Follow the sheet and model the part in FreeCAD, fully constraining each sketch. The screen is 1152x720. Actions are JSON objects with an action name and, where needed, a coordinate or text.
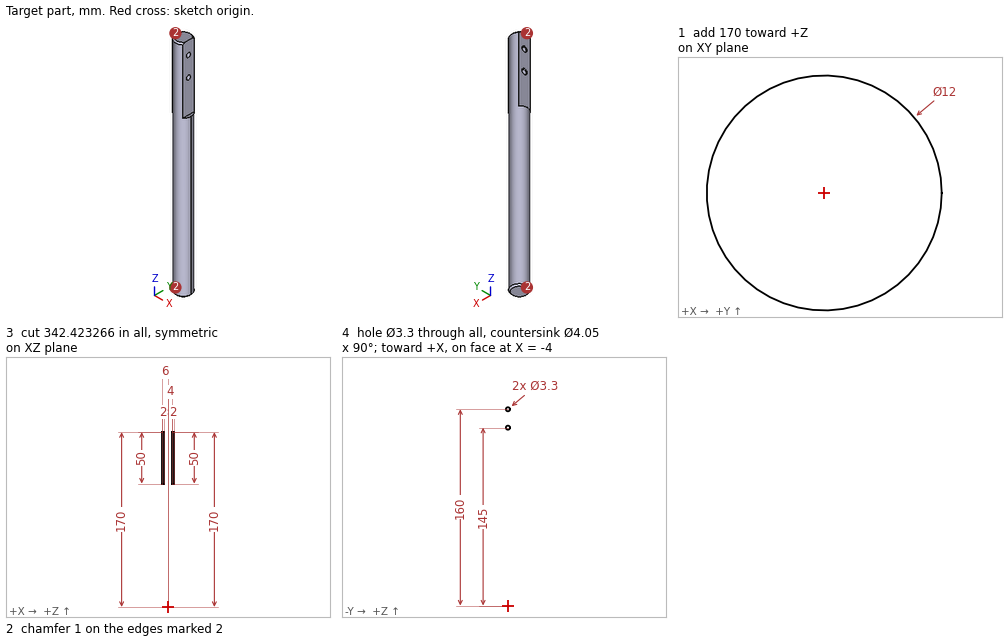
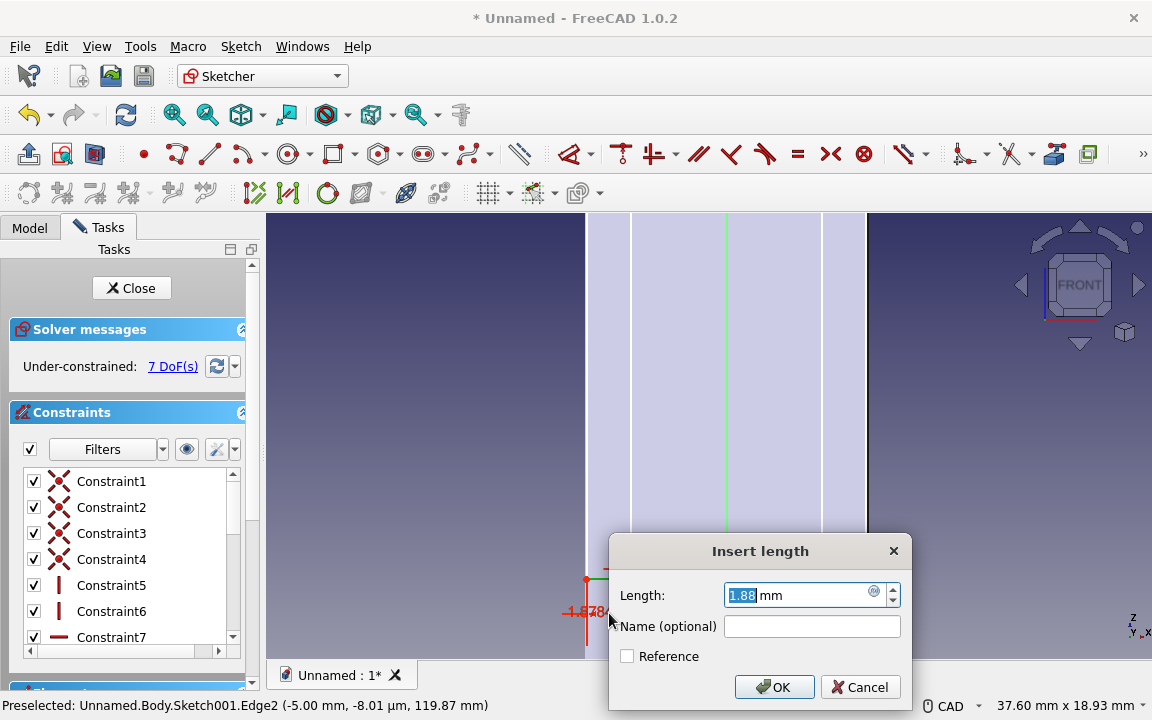
{"action": "type", "text": "2"}
{"action": "key", "text": "Return"}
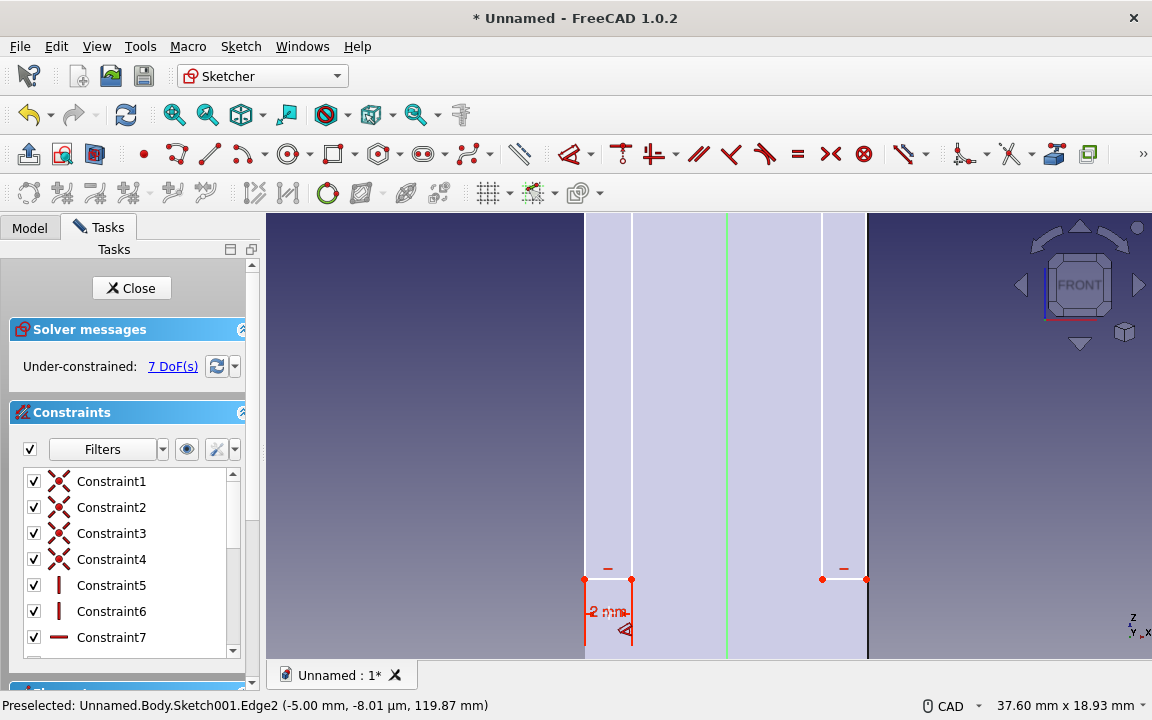
{"action": "left_click", "coordinate": [835, 579]}
{"action": "left_click", "coordinate": [844, 613]}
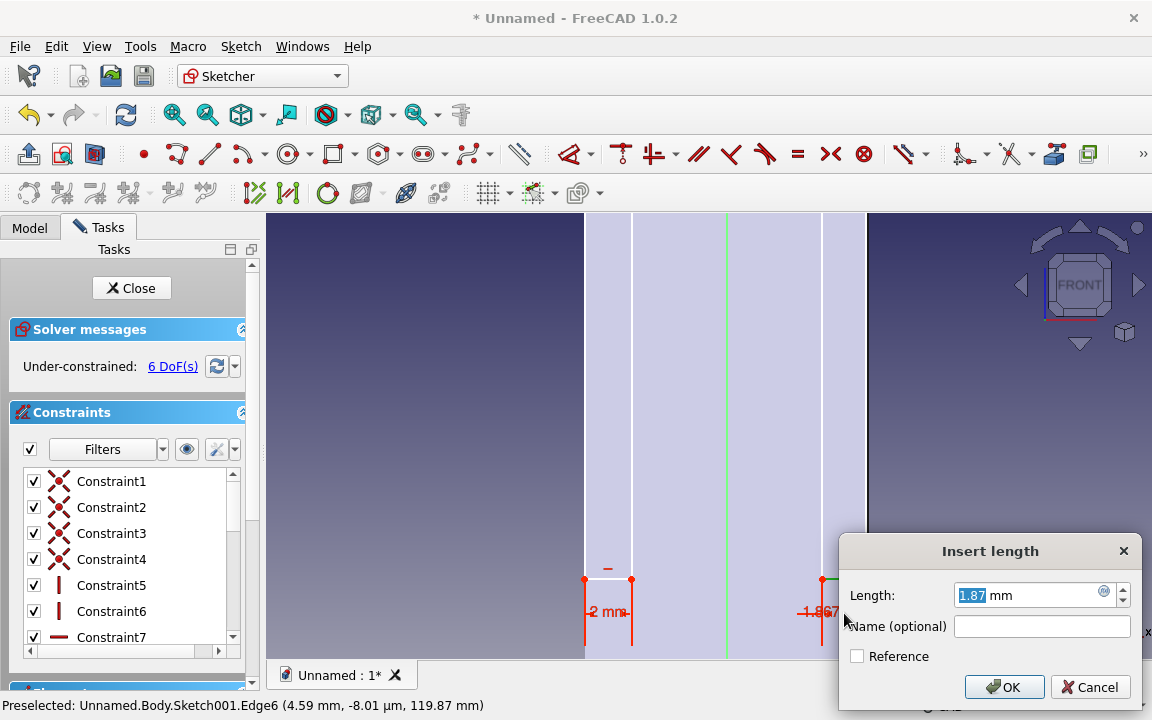
{"action": "type", "text": "2"}
{"action": "key", "text": "Return"}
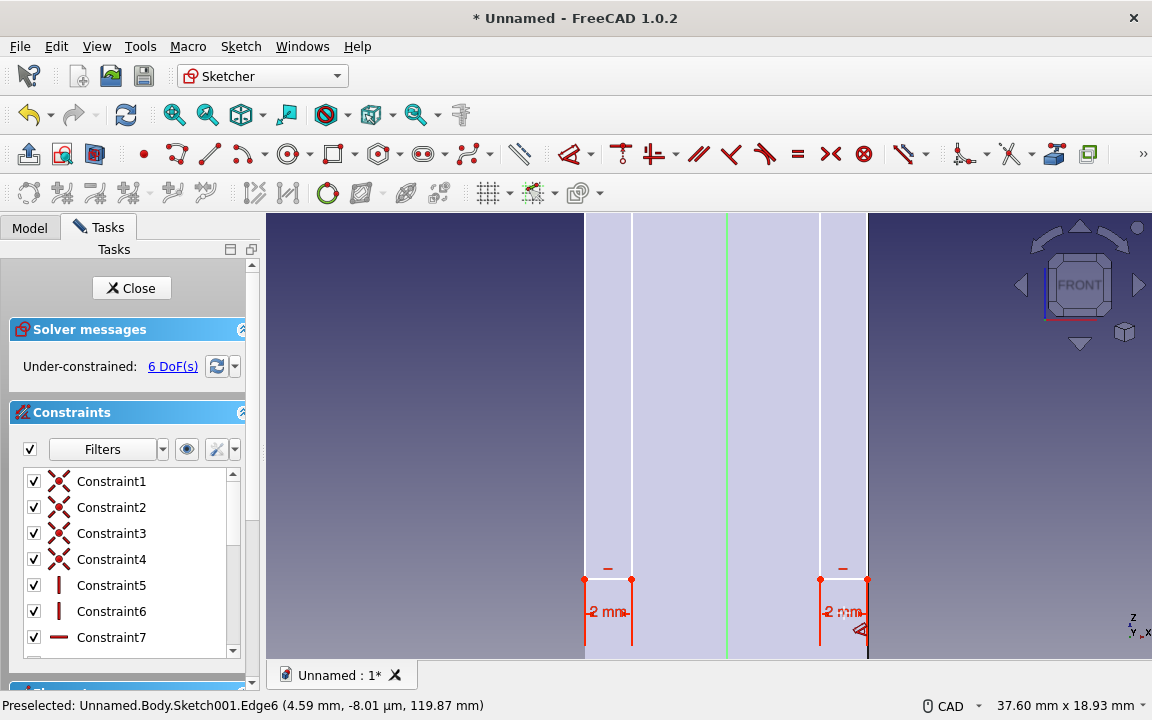
{"action": "scroll", "coordinate": [612, 583], "scroll_direction": "down", "scroll_amount": 7}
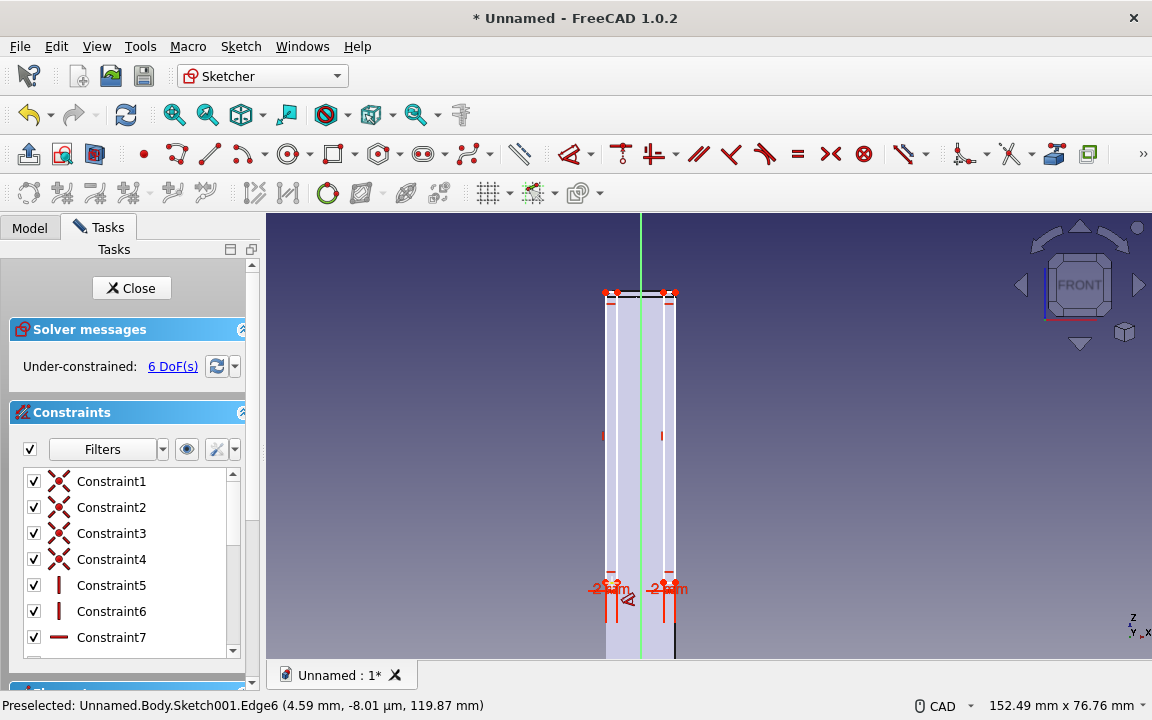
{"action": "left_click", "coordinate": [606, 525]}
{"action": "left_click", "coordinate": [572, 438]}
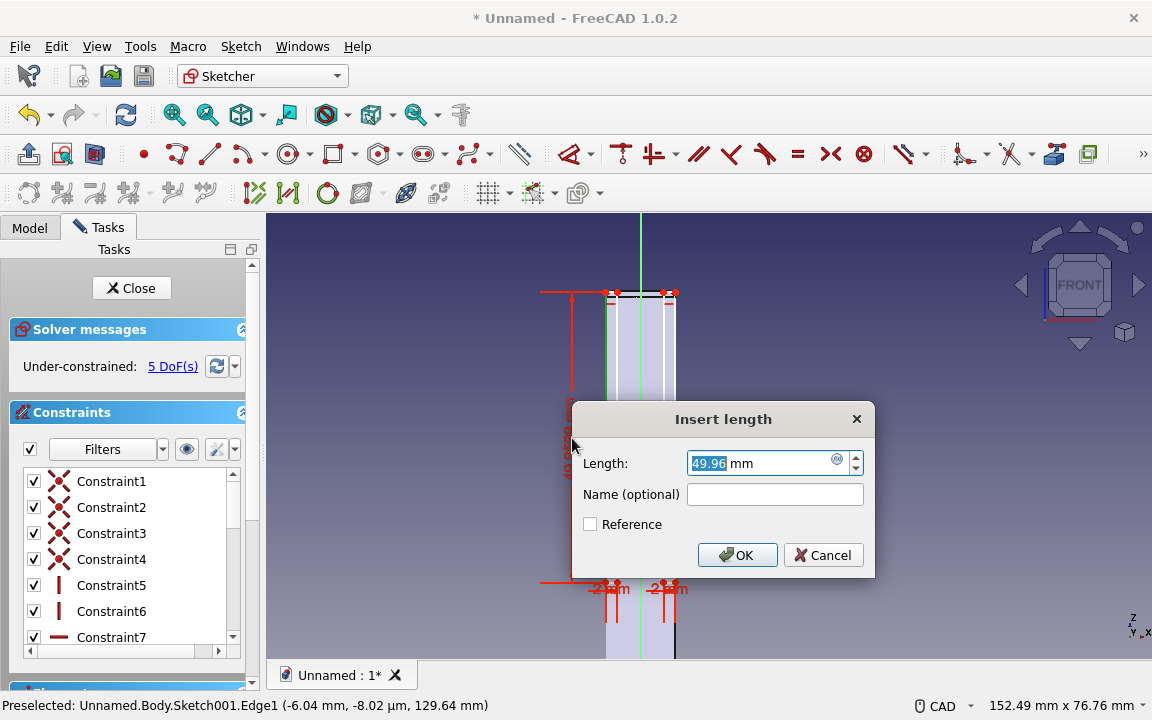
{"action": "type", "text": "50"}
{"action": "key", "text": "Return"}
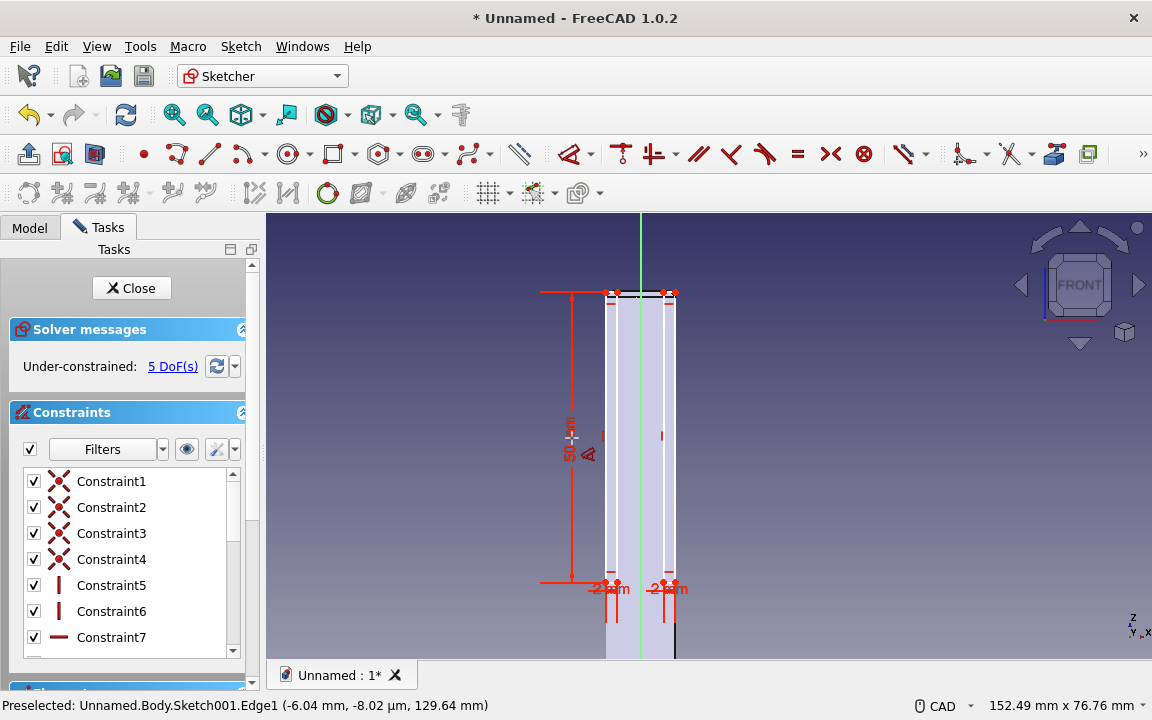
{"action": "left_click", "coordinate": [664, 380]}
{"action": "left_click", "coordinate": [698, 438]}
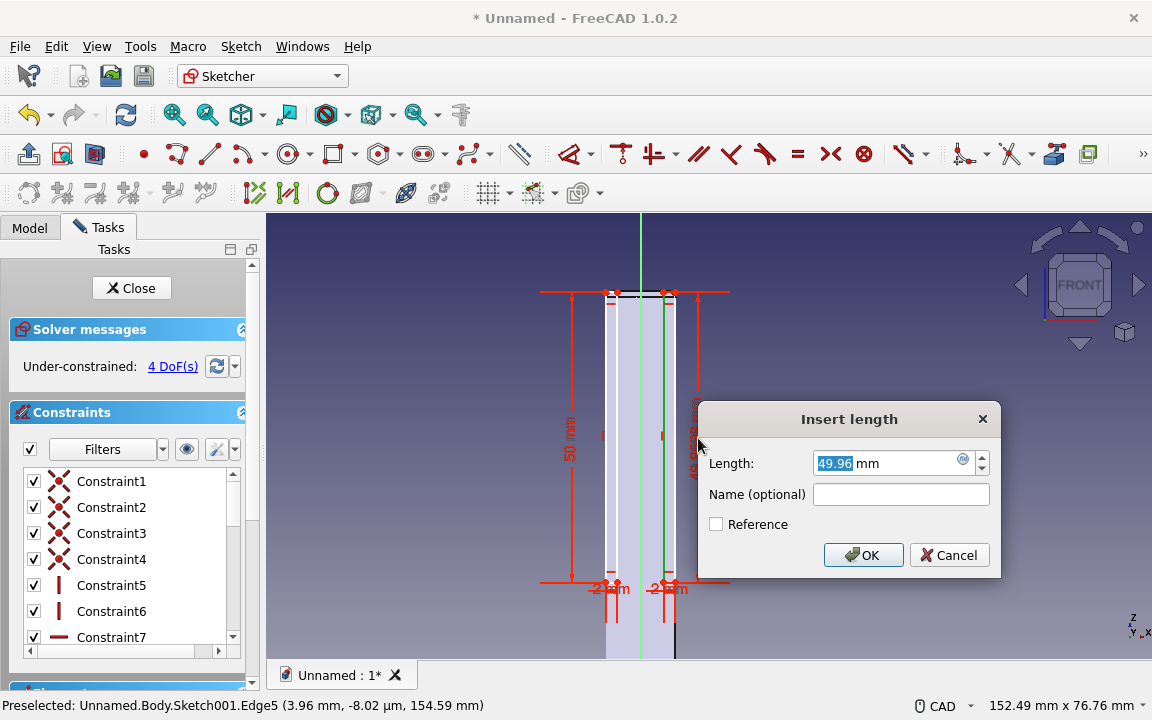
{"action": "type", "text": "50"}
{"action": "key", "text": "Return"}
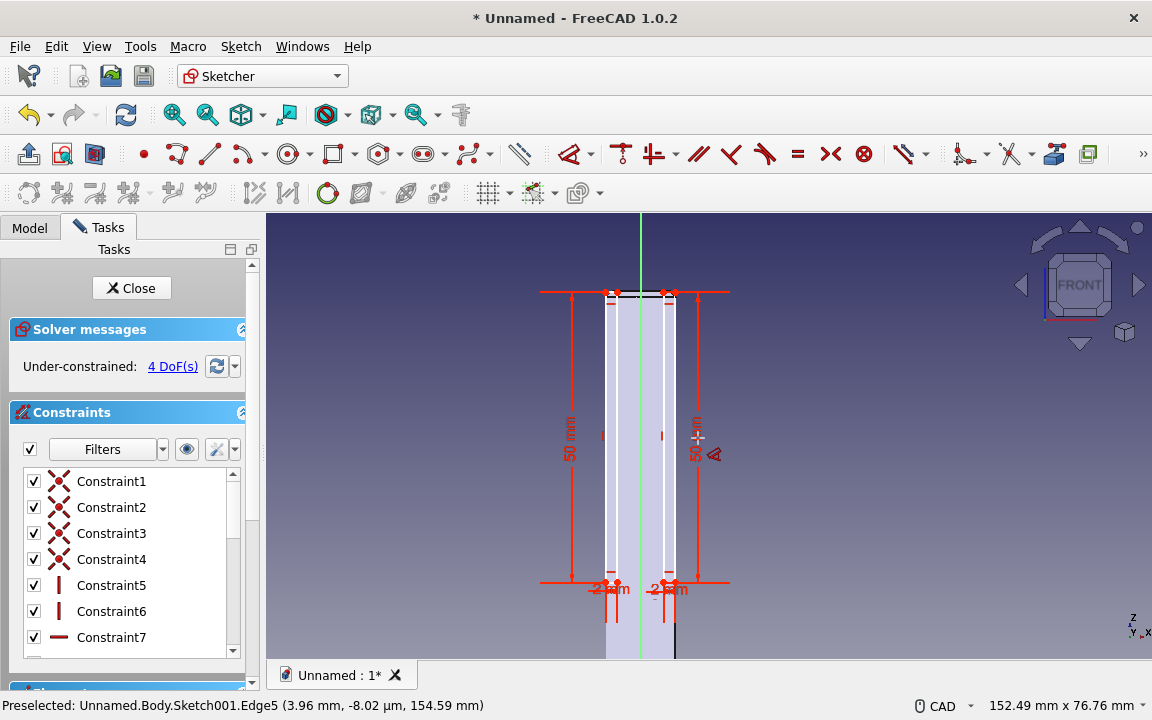
{"action": "left_click", "coordinate": [606, 292]}
{"action": "left_click", "coordinate": [623, 258]}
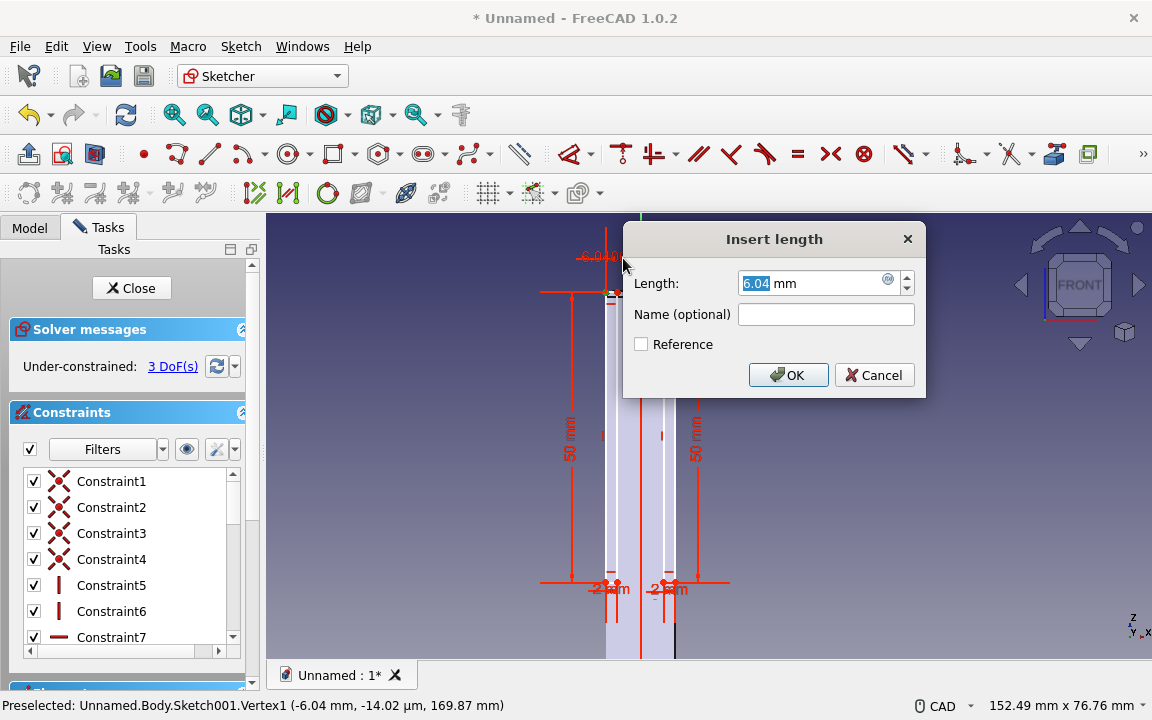
{"action": "type", "text": "6"}
{"action": "key", "text": "Return"}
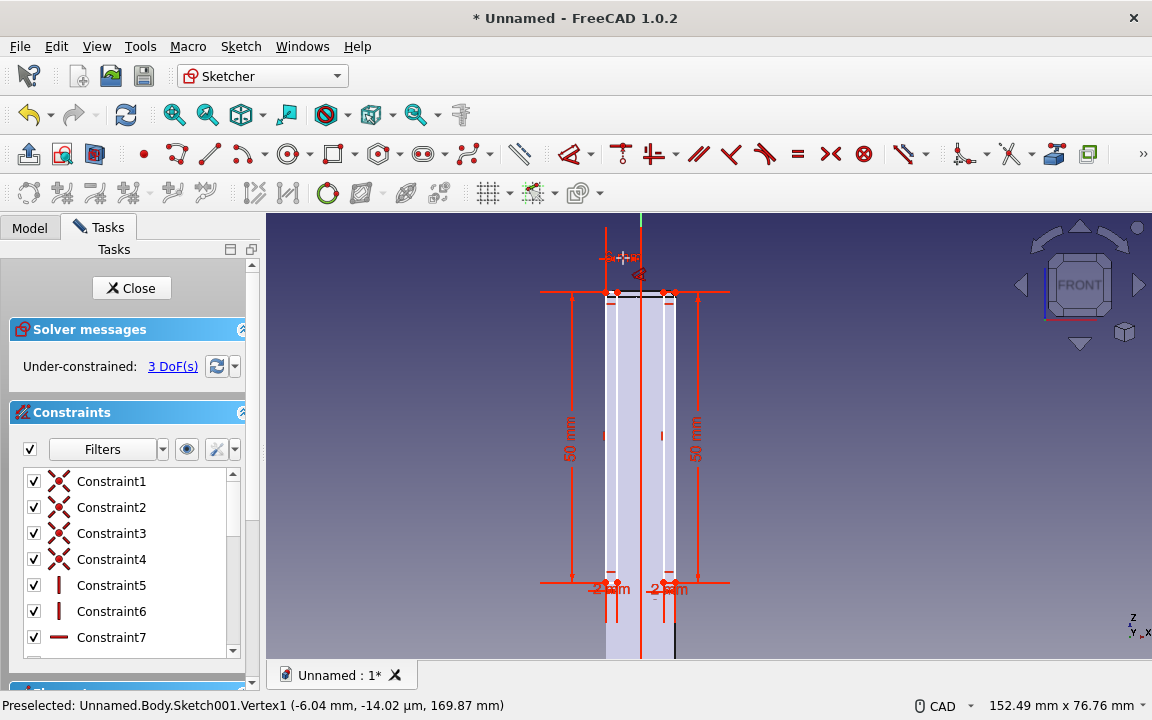
{"action": "scroll", "coordinate": [664, 292], "scroll_direction": "up", "scroll_amount": 3}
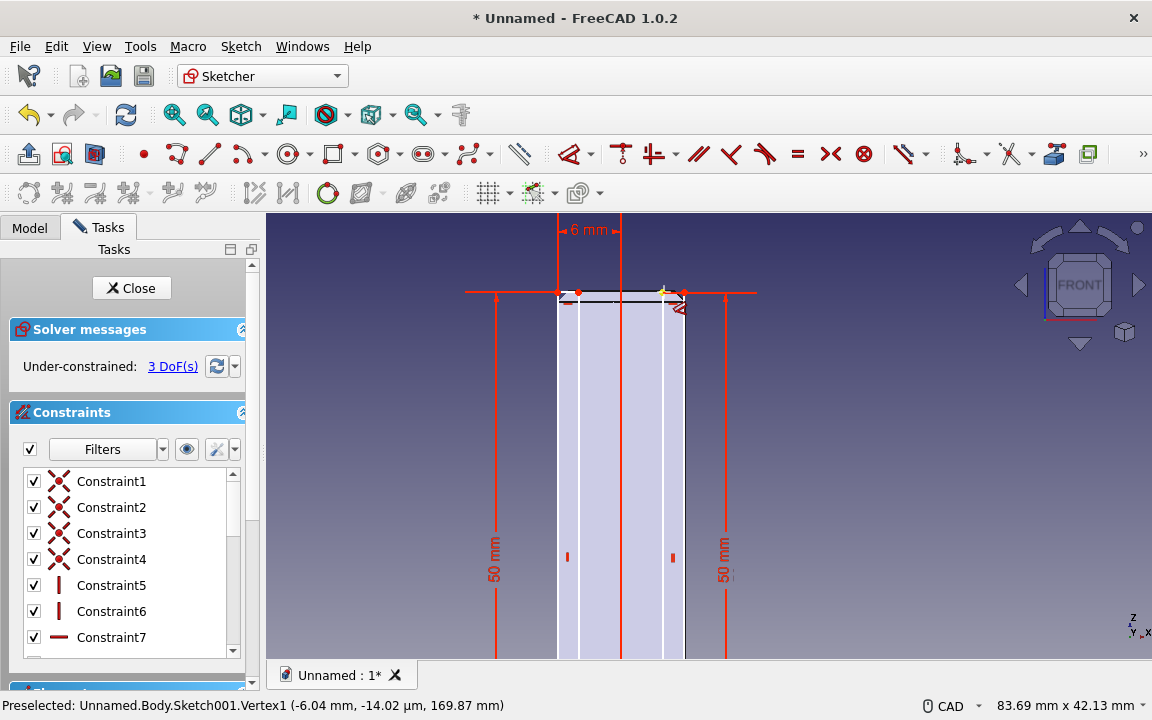
{"action": "left_click", "coordinate": [663, 293]}
{"action": "left_click", "coordinate": [642, 259]}